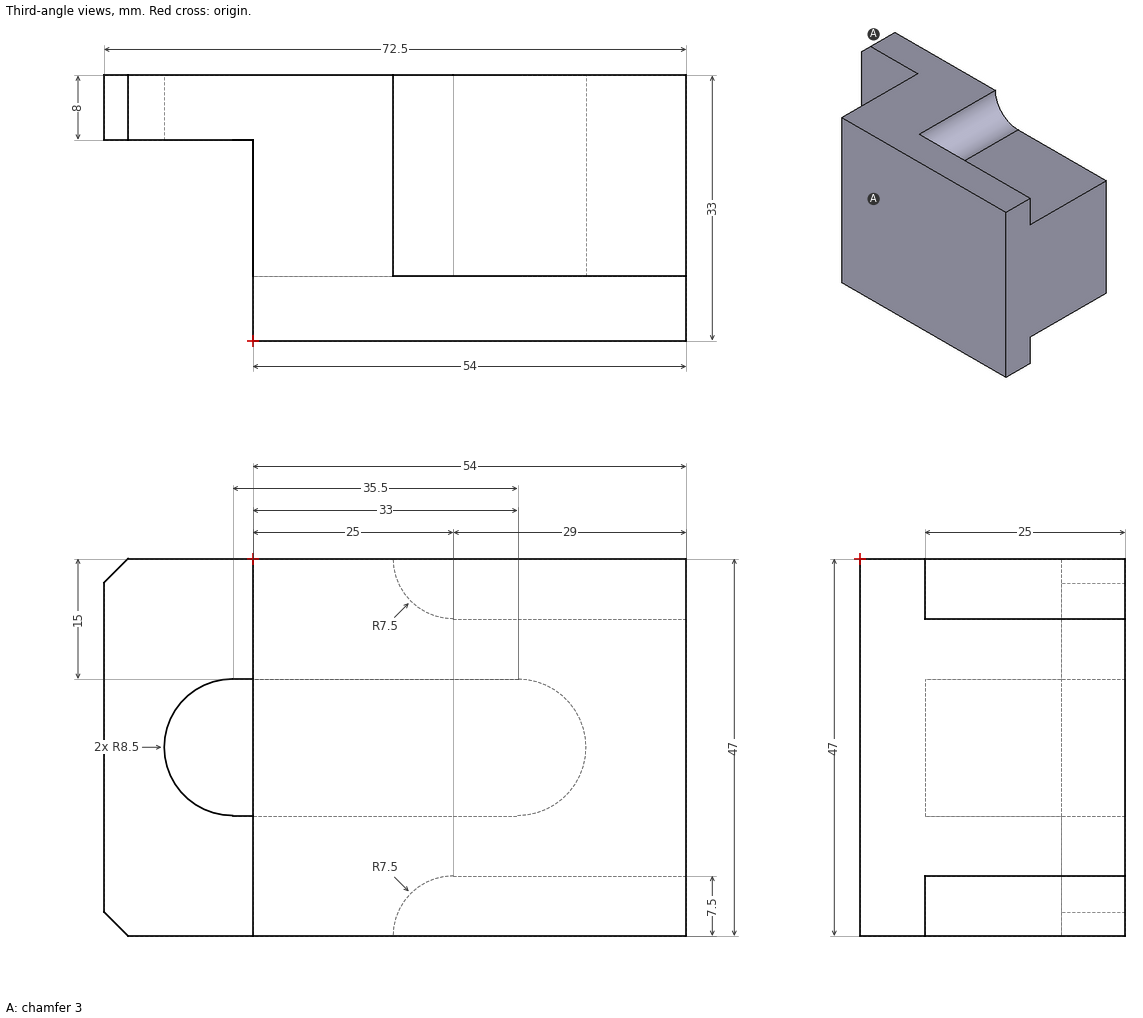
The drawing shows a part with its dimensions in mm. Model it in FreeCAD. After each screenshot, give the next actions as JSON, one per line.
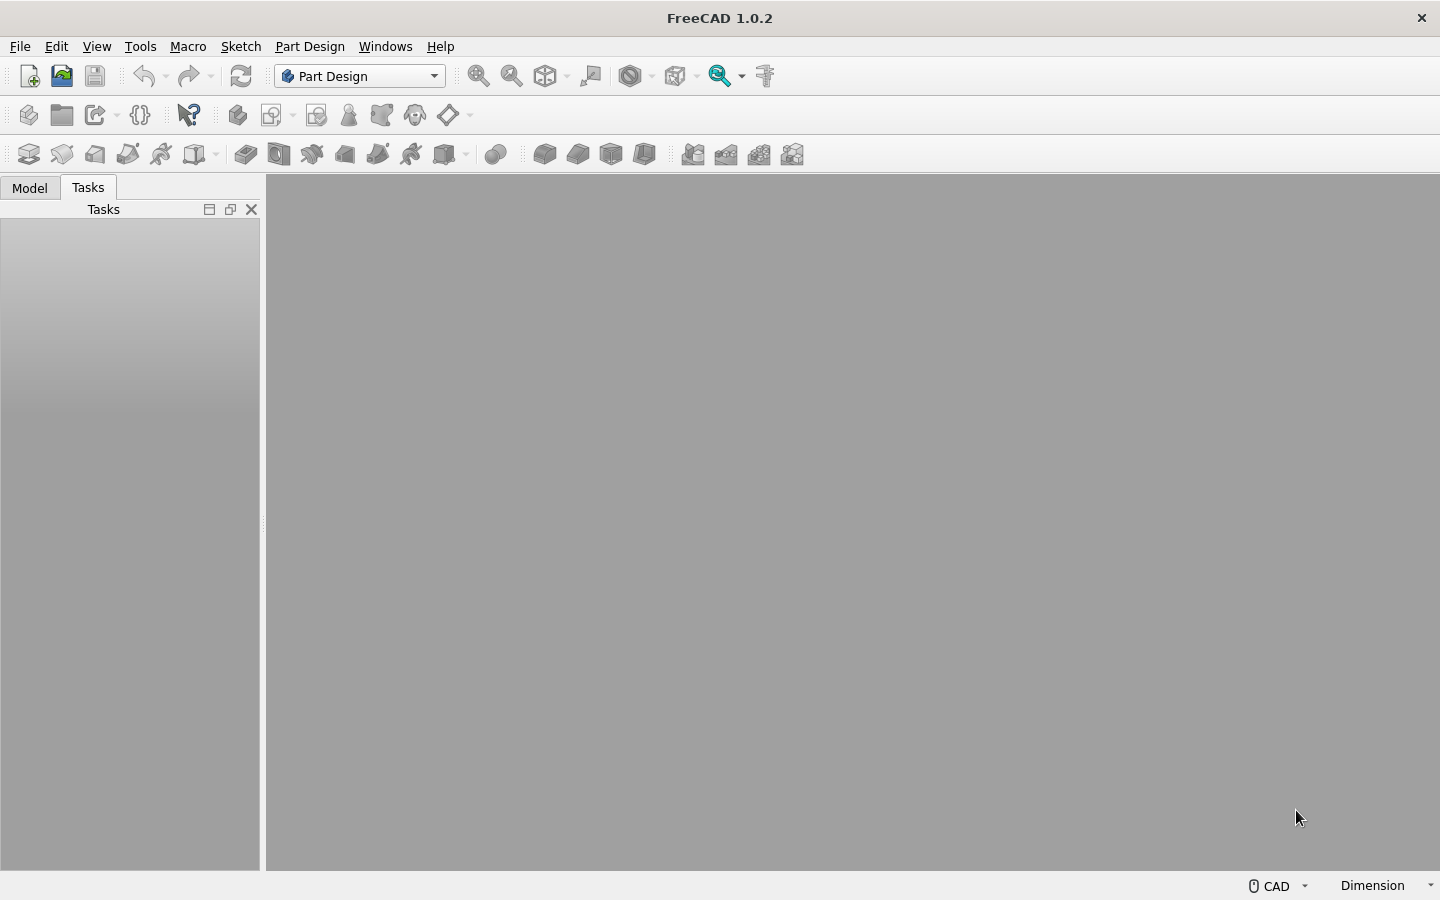
{"action": "left_click", "coordinate": [29, 76]}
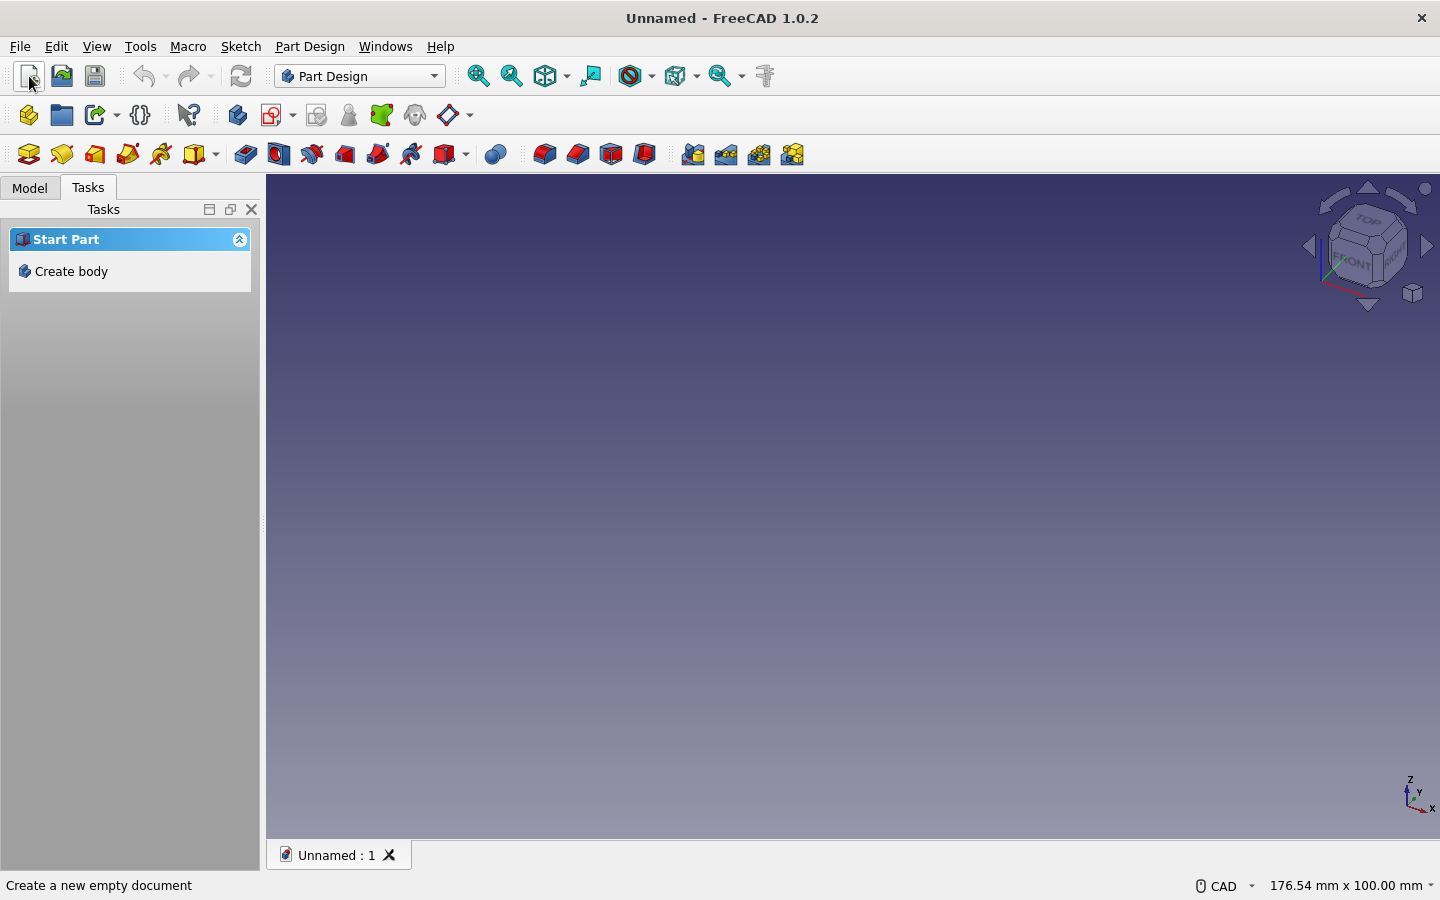
{"action": "left_click", "coordinate": [270, 116]}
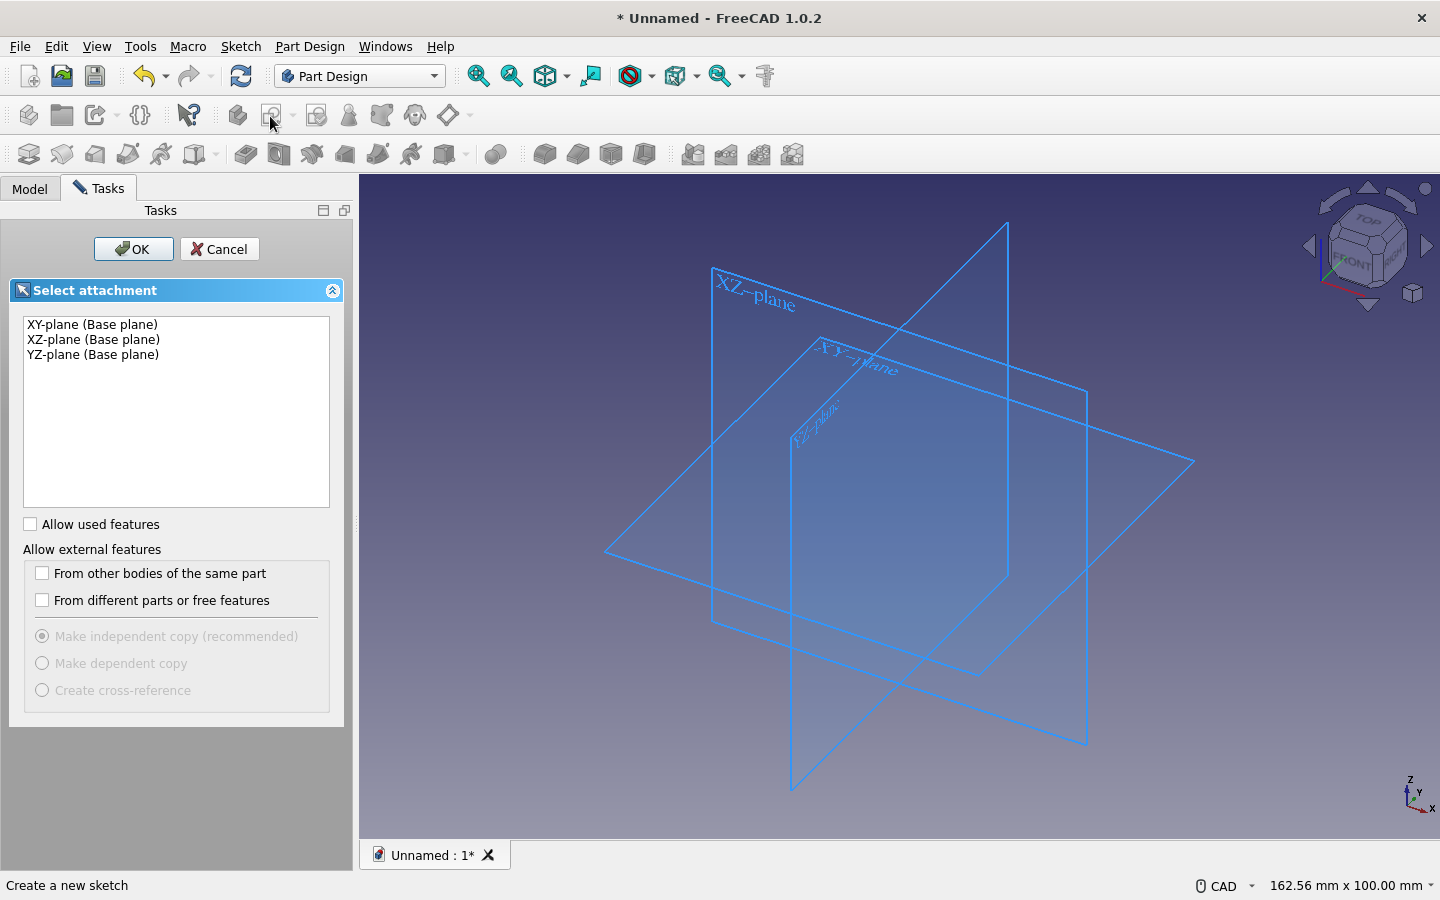
{"action": "left_click", "coordinate": [84, 324]}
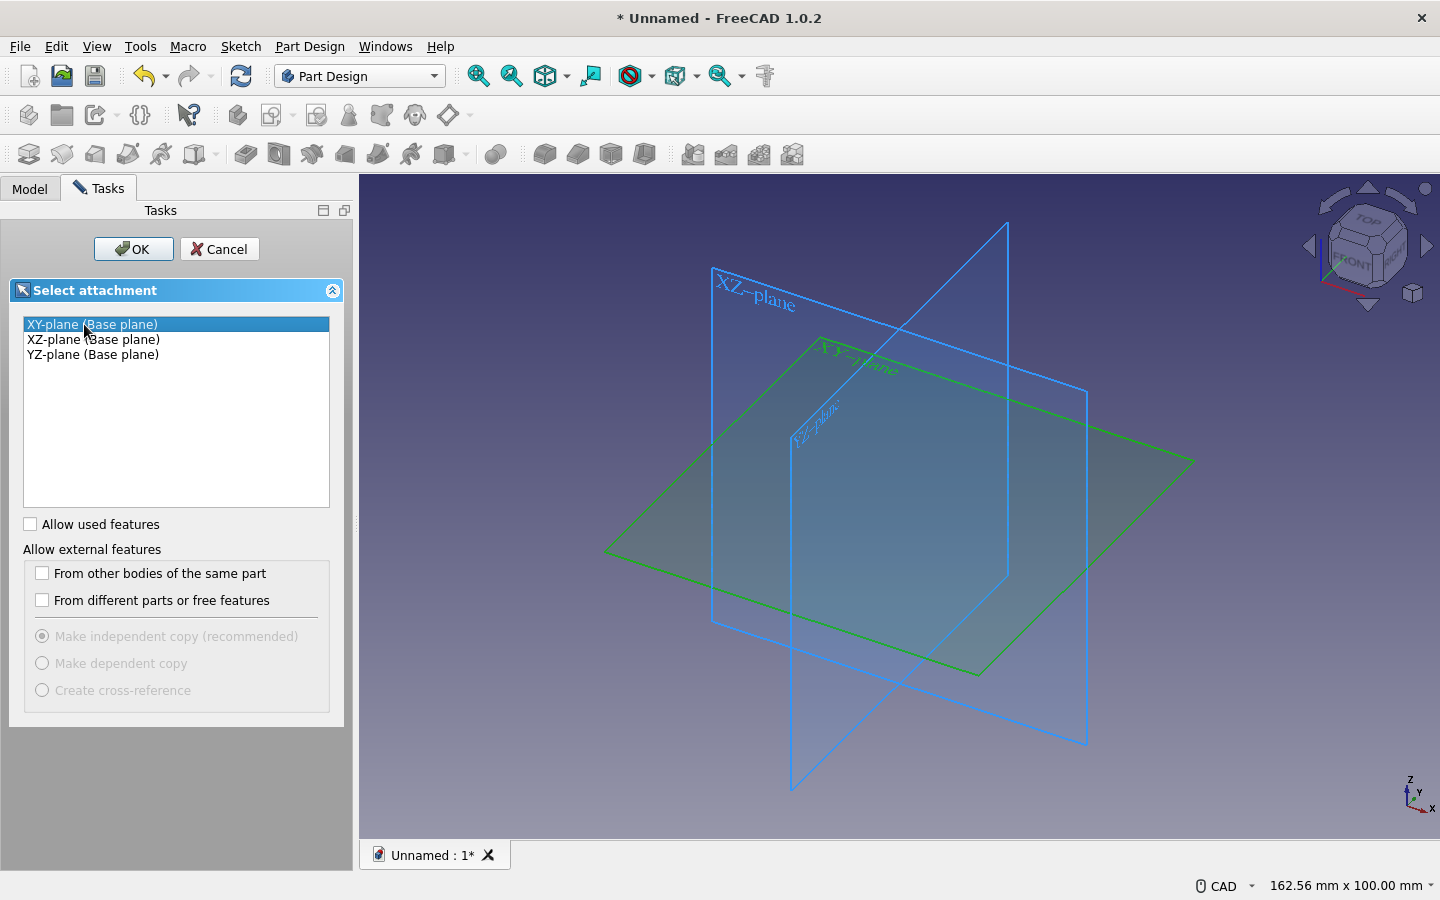
{"action": "left_click", "coordinate": [134, 249]}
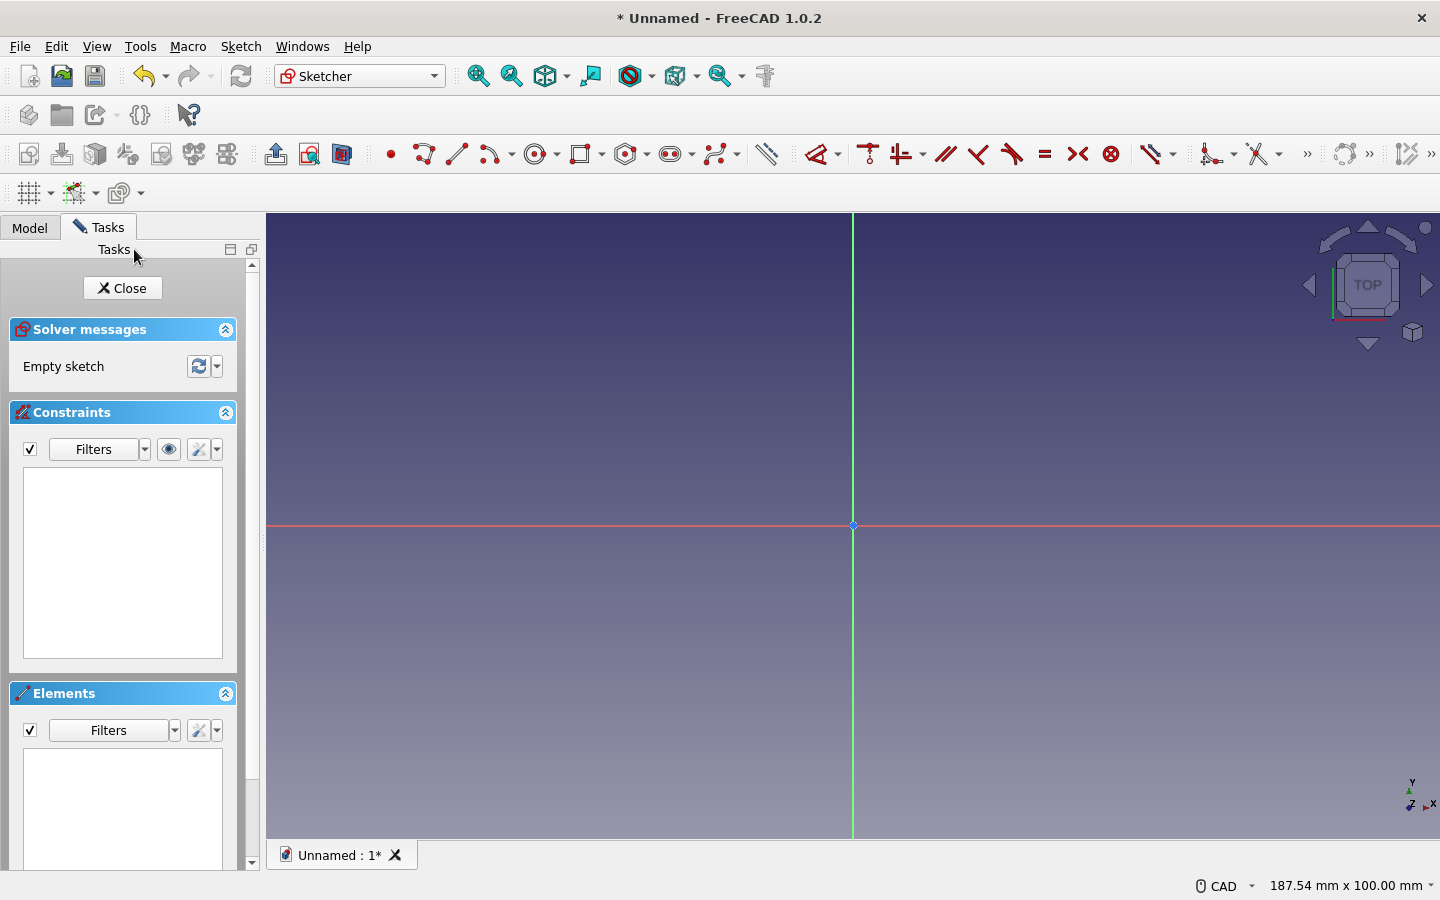
{"action": "scroll", "coordinate": [1275, 241], "scroll_direction": "up", "scroll_amount": 2}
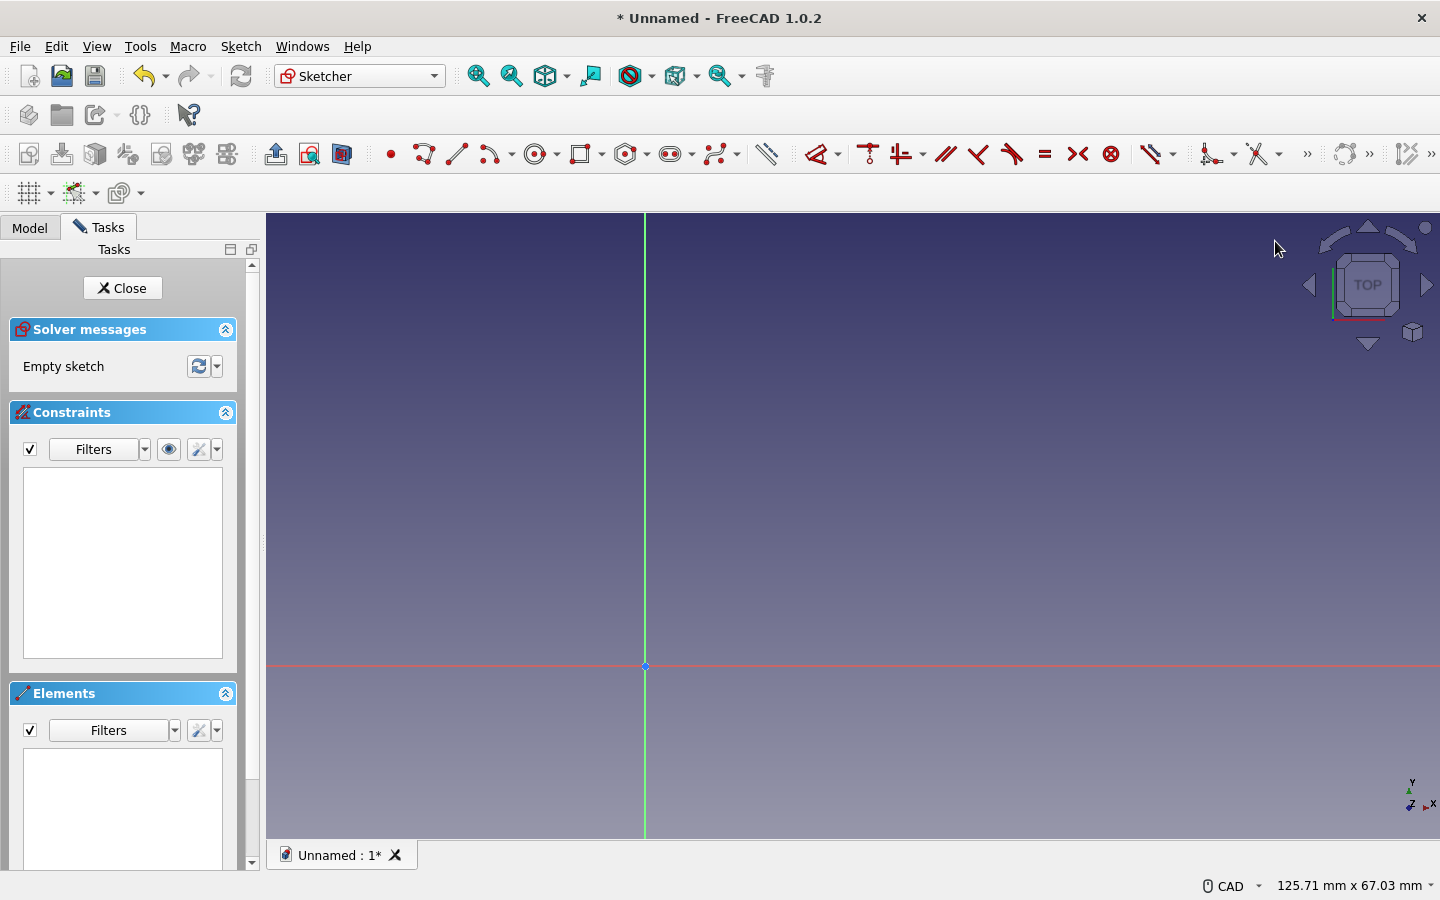
{"action": "key", "text": "g m"}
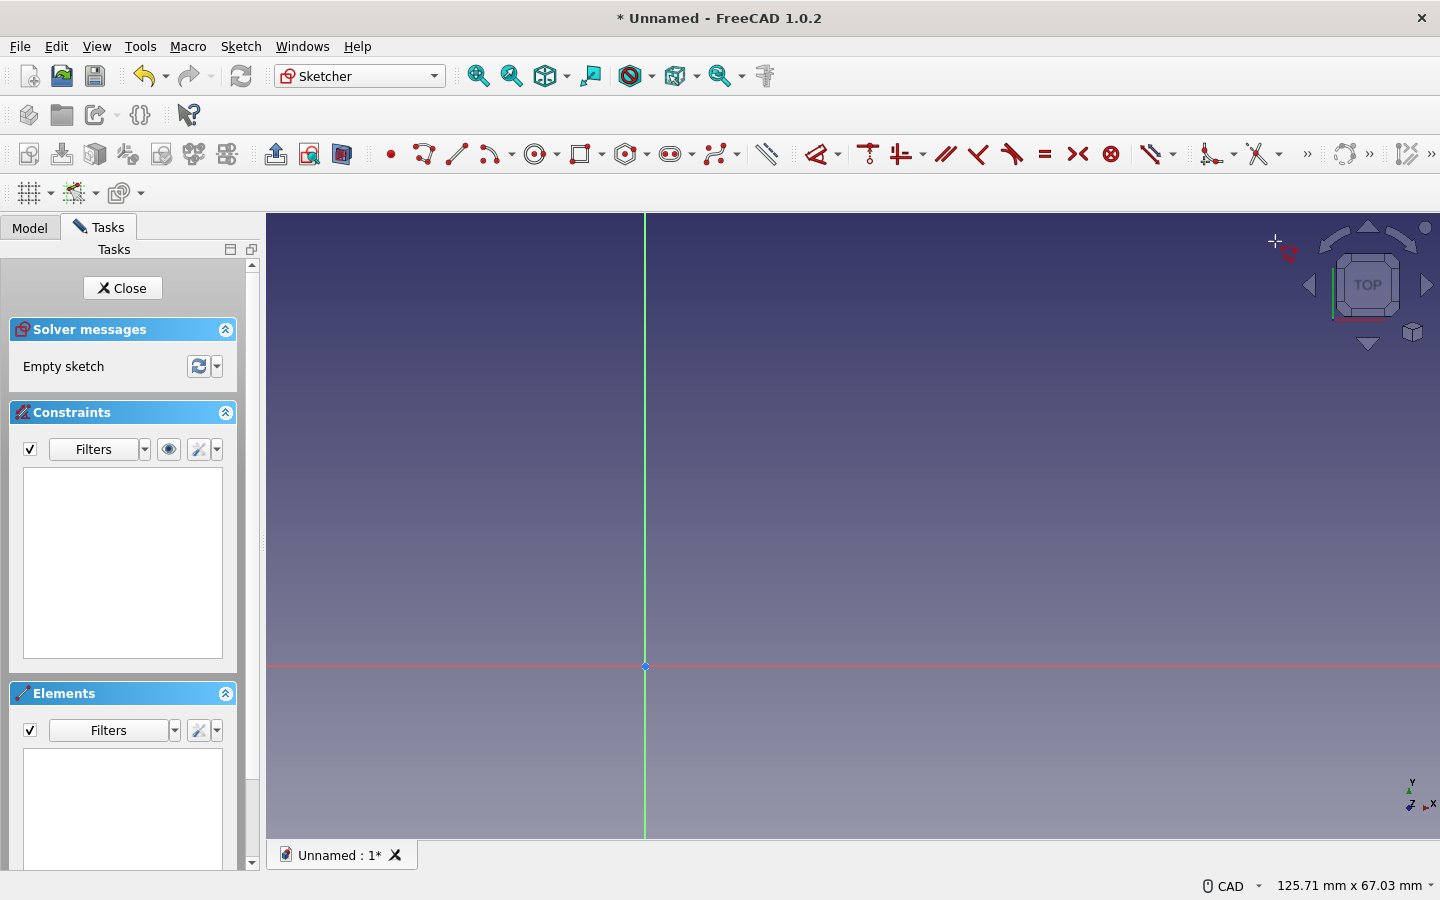
{"action": "left_click", "coordinate": [645, 666]}
{"action": "left_click", "coordinate": [1149, 657]}
{"action": "left_click", "coordinate": [1149, 358]}
{"action": "left_click", "coordinate": [472, 358]}
{"action": "left_click", "coordinate": [472, 433]}
{"action": "left_click", "coordinate": [654, 433]}
{"action": "left_click", "coordinate": [645, 666]}
{"action": "key", "text": "Escape"}
{"action": "key", "text": "Escape"}